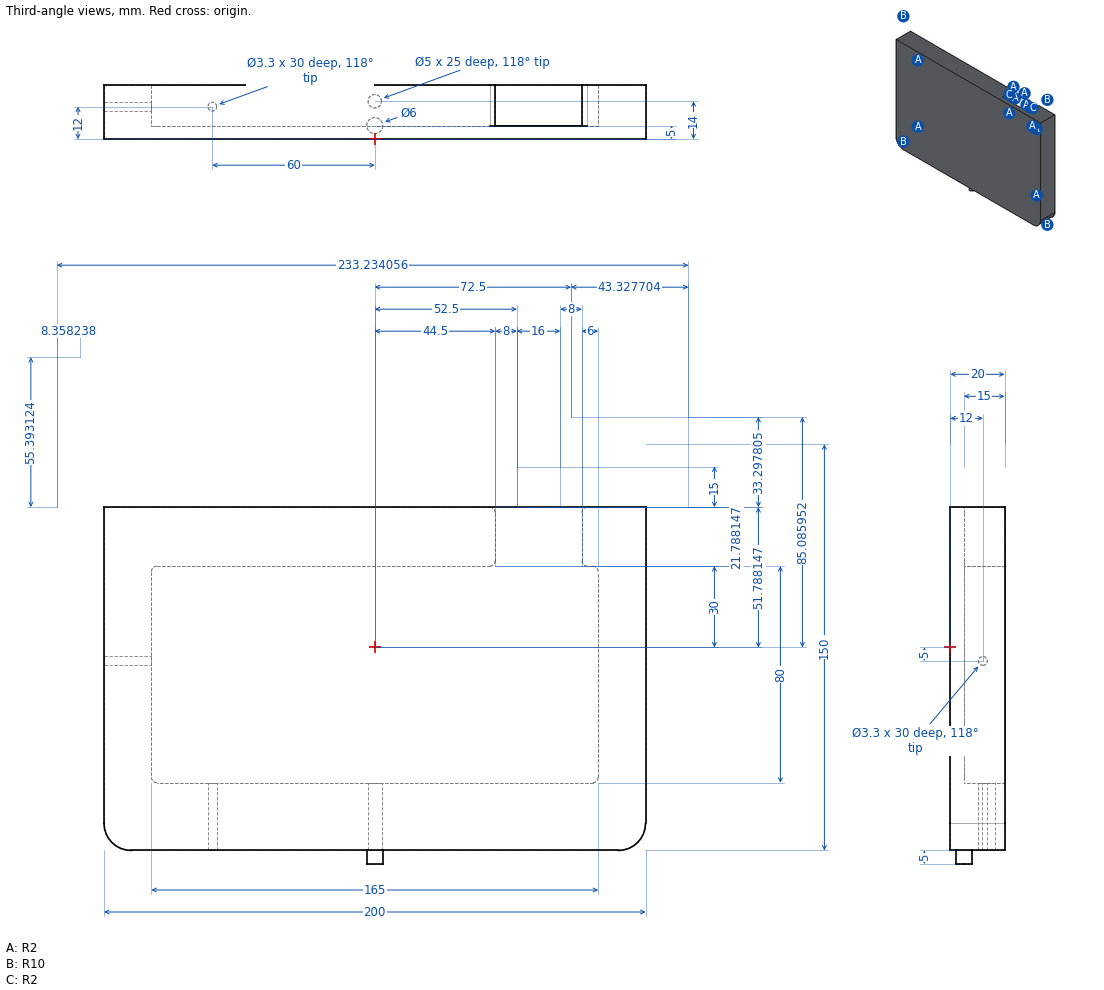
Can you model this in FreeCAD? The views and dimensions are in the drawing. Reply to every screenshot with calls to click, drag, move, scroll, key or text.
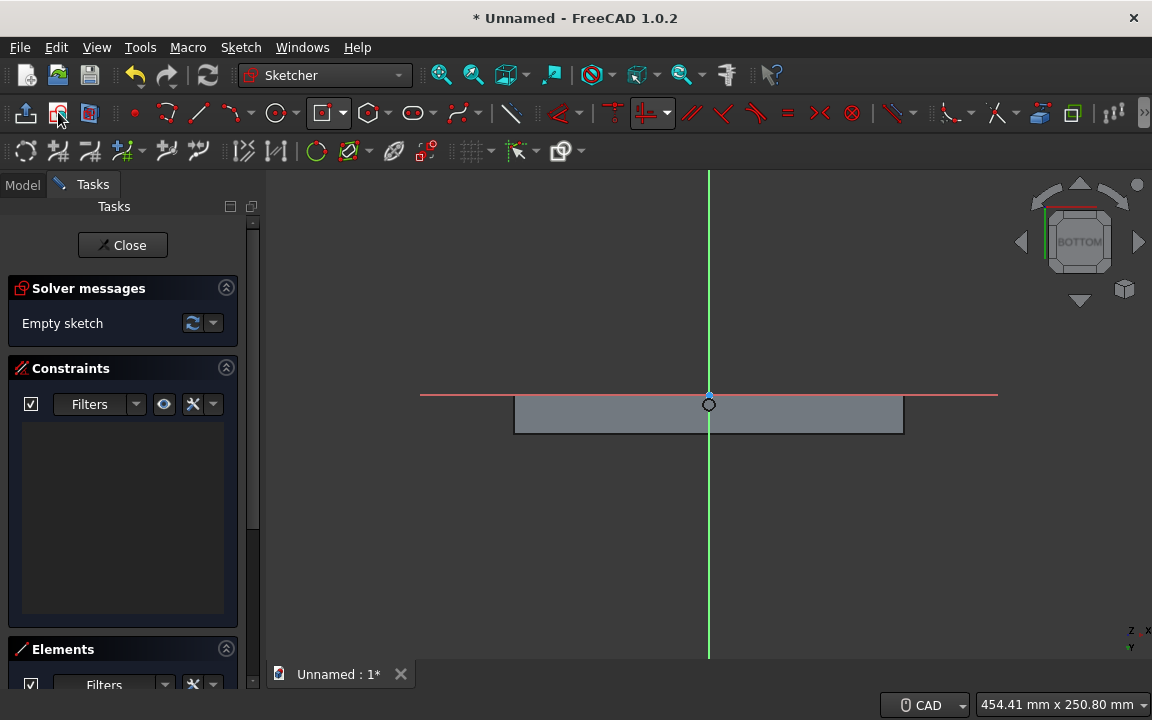
key(q)
key(s)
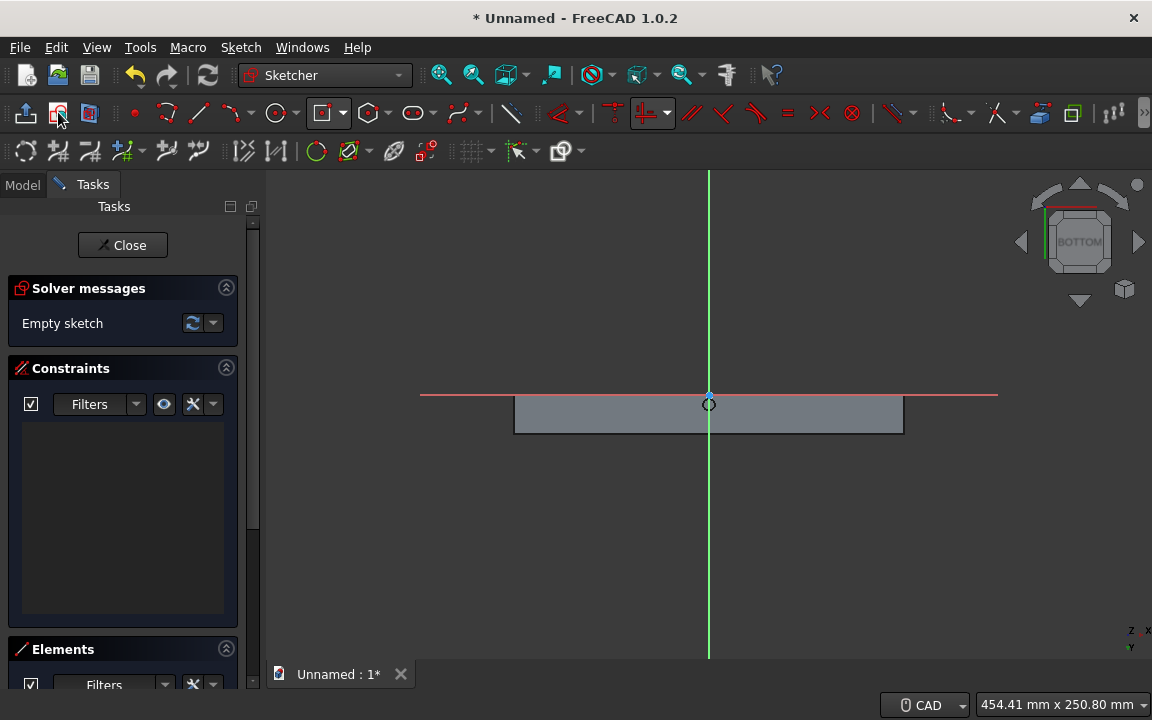
scroll(713, 423, up, 15)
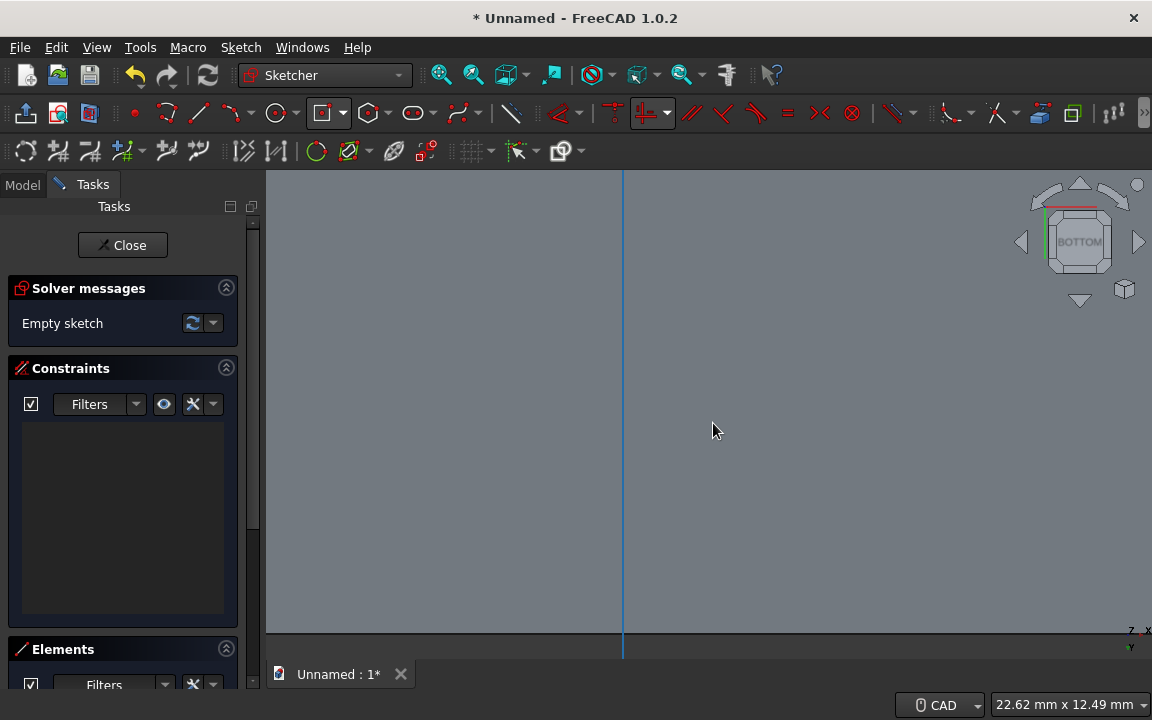
scroll(587, 368, up, 2)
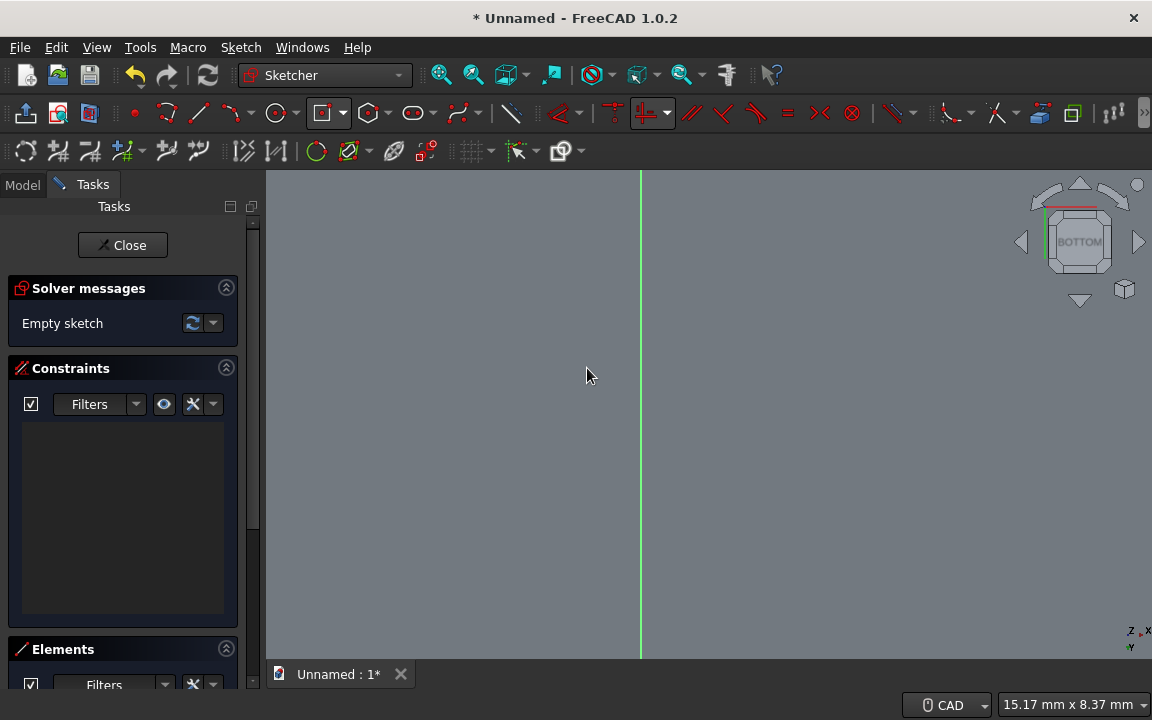
click(276, 114)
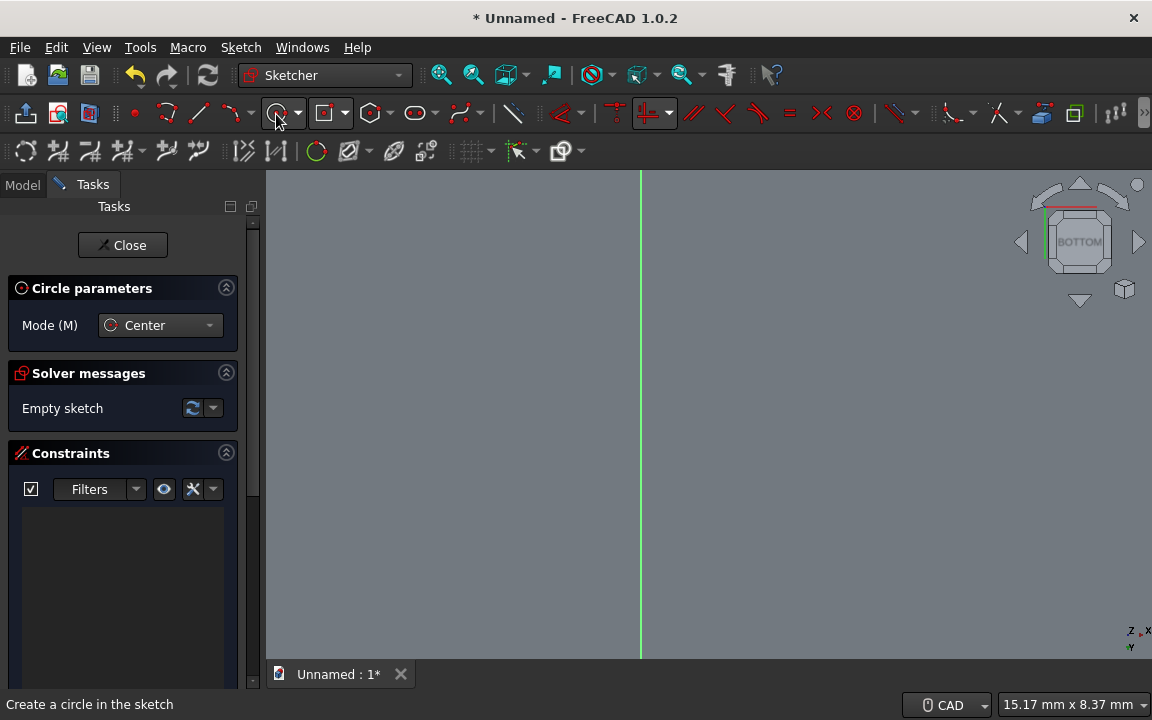
click(641, 414)
click(744, 311)
key(Escape)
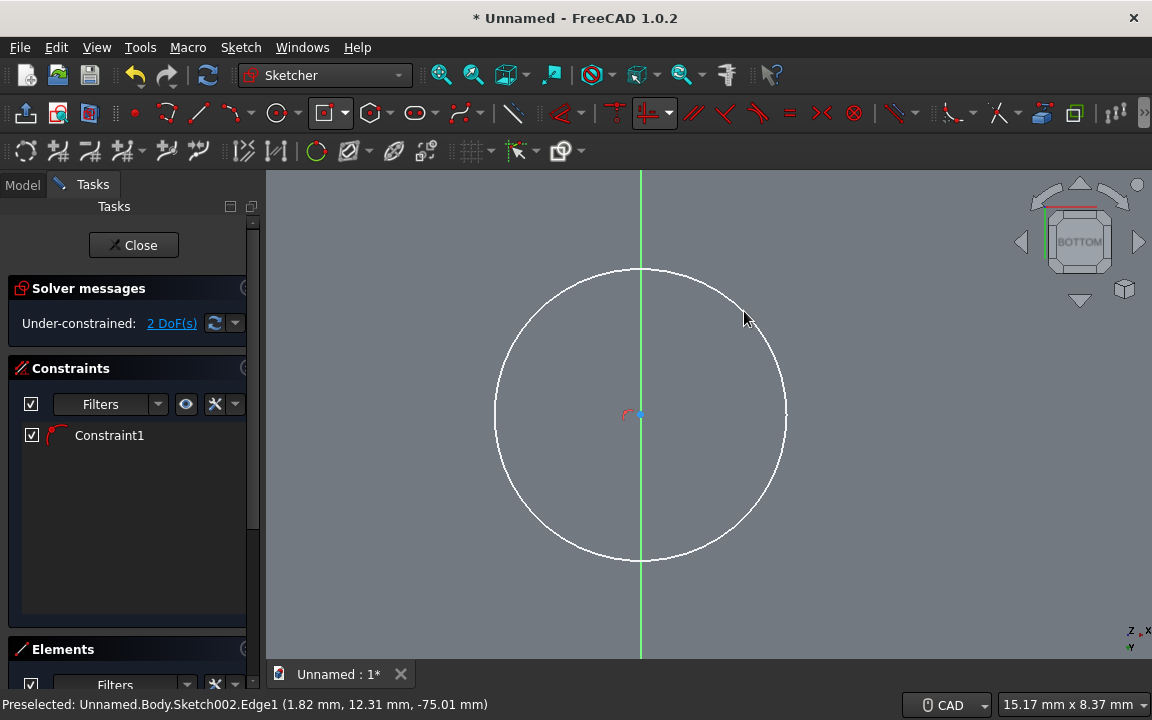
key(d)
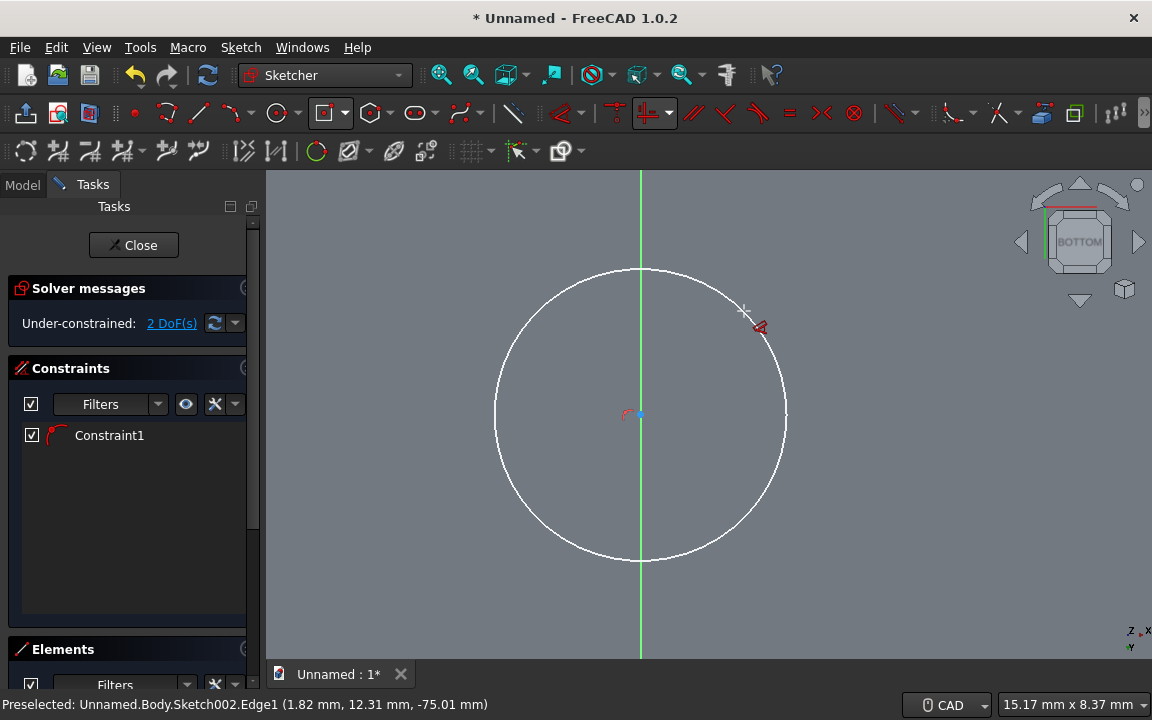
click(743, 311)
click(765, 288)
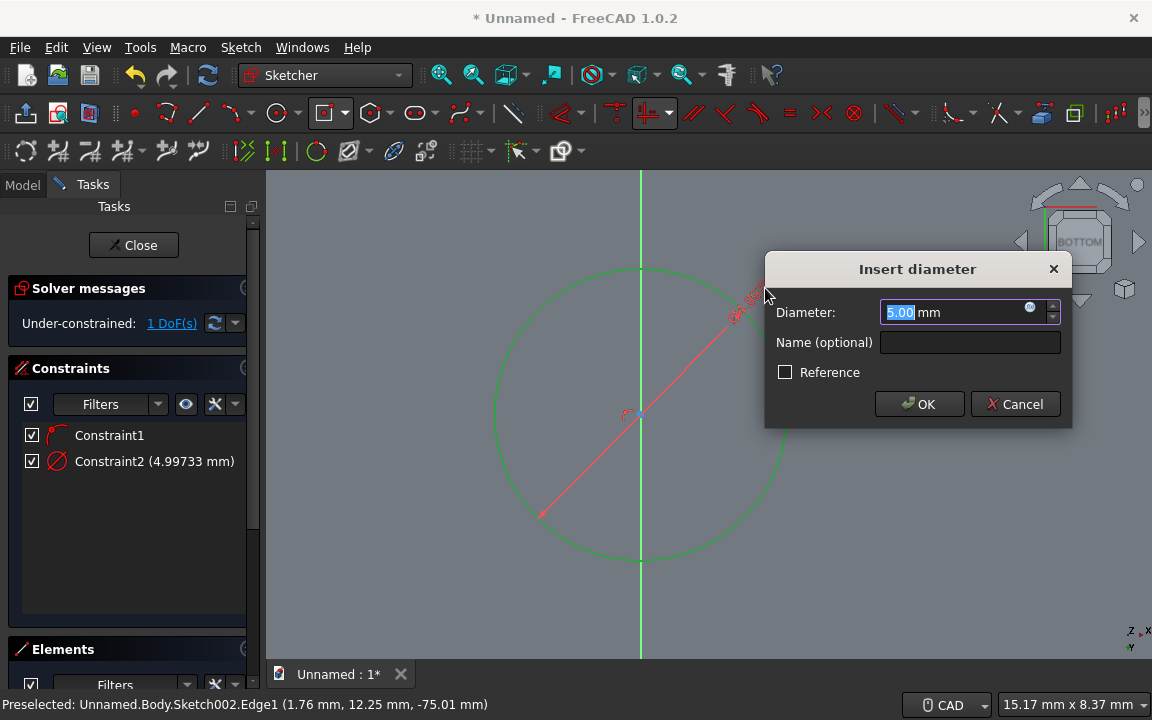
text(5)
key(Return)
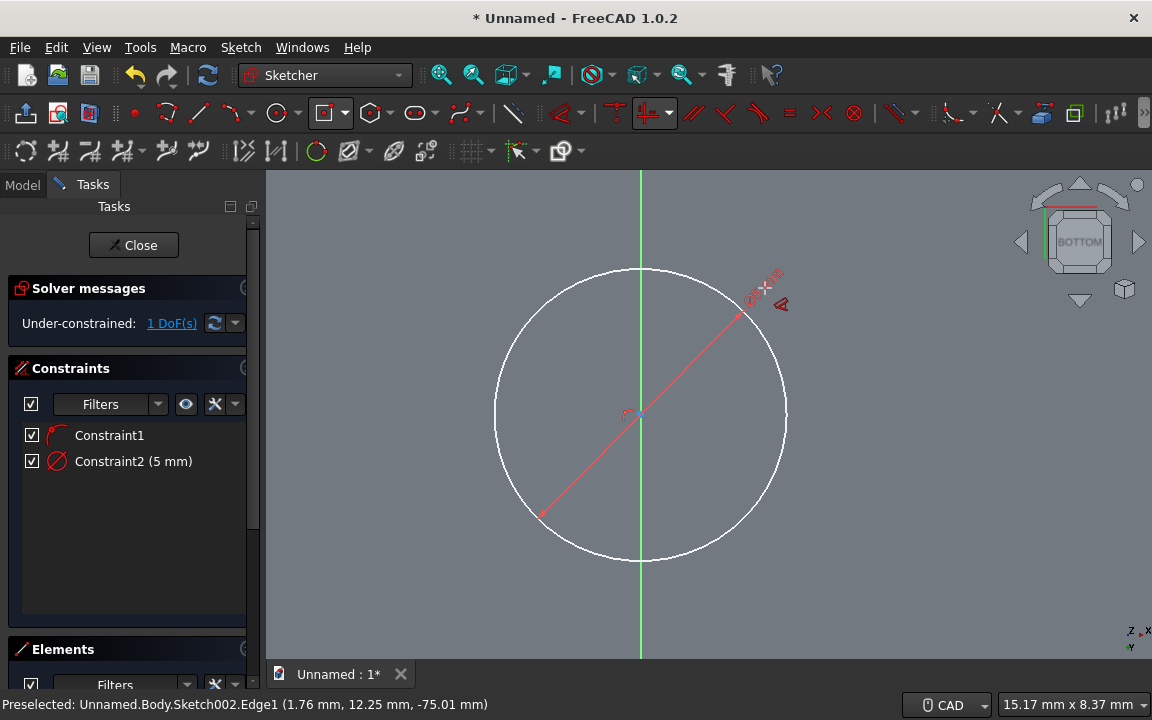
click(641, 415)
click(675, 307)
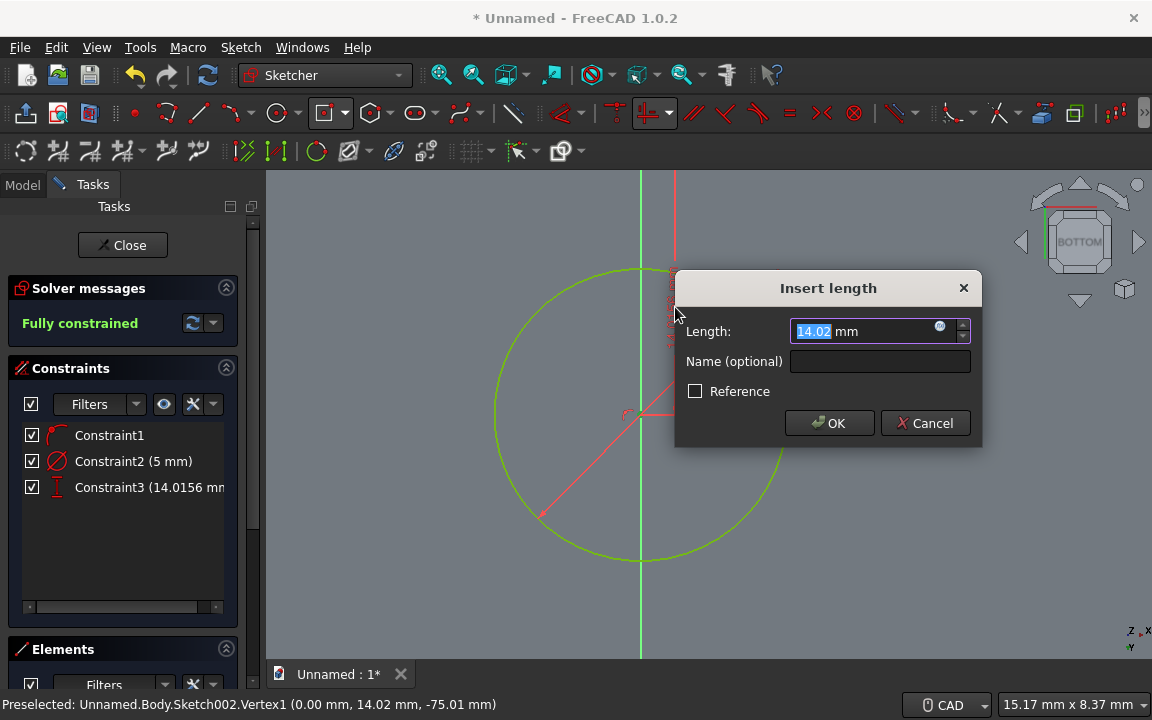
text(14)
key(Return)
key(Escape)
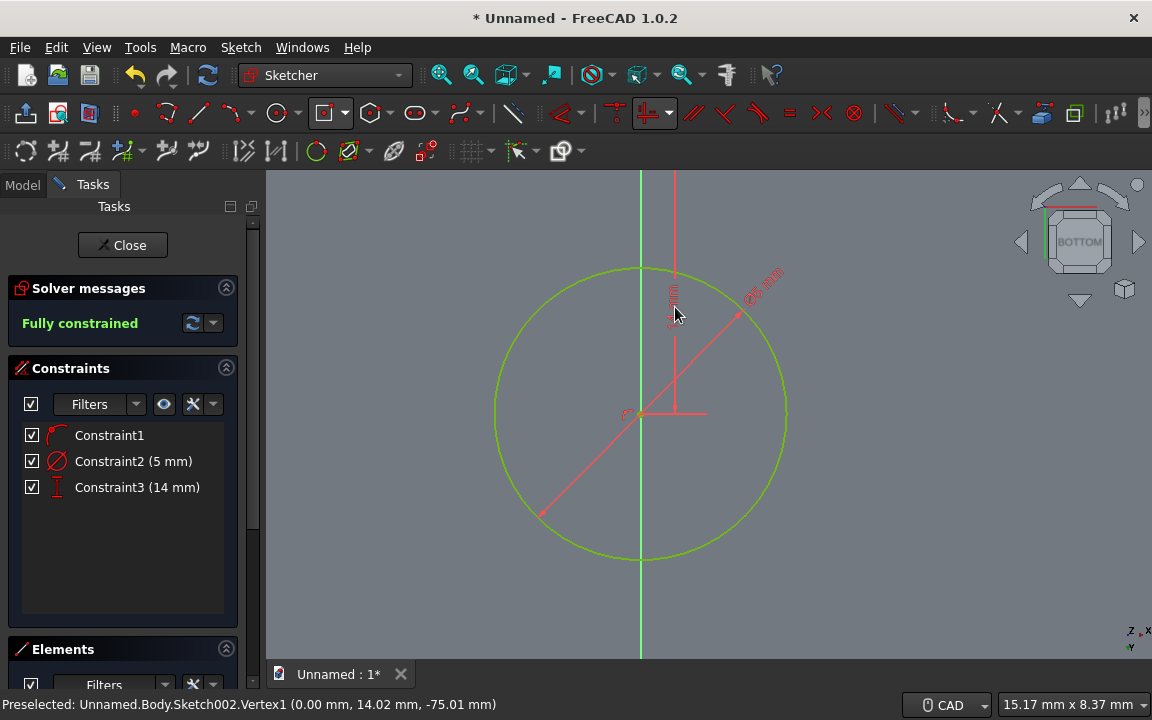
click(123, 245)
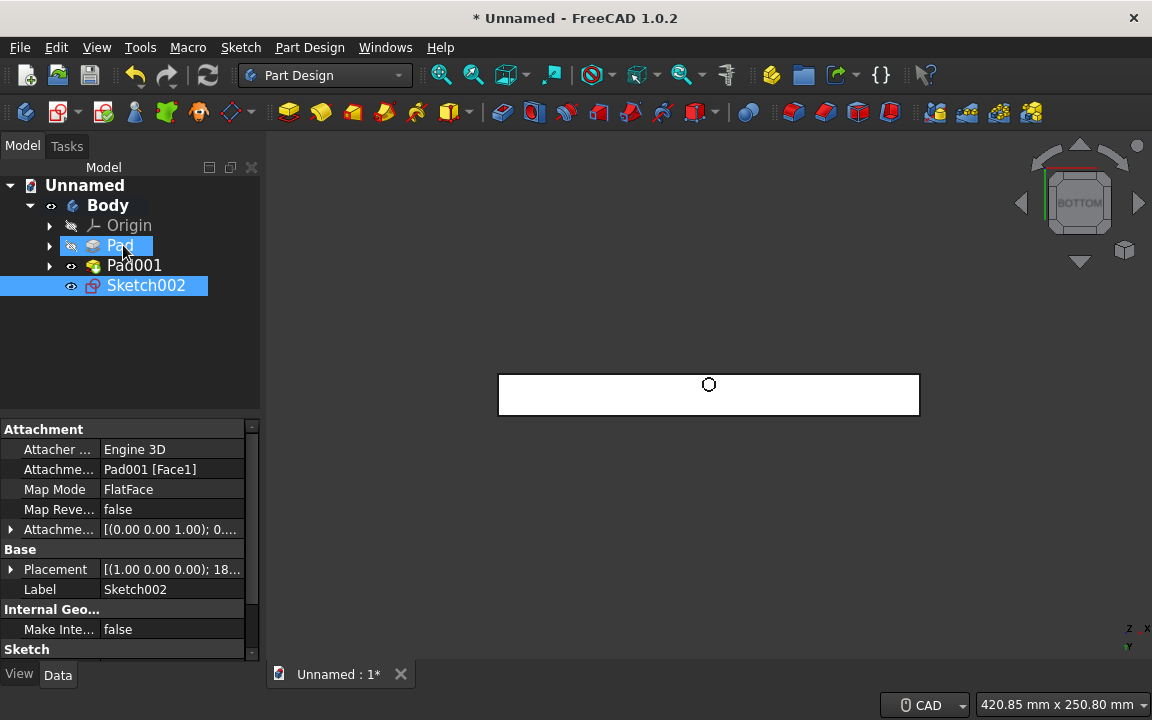
click(536, 112)